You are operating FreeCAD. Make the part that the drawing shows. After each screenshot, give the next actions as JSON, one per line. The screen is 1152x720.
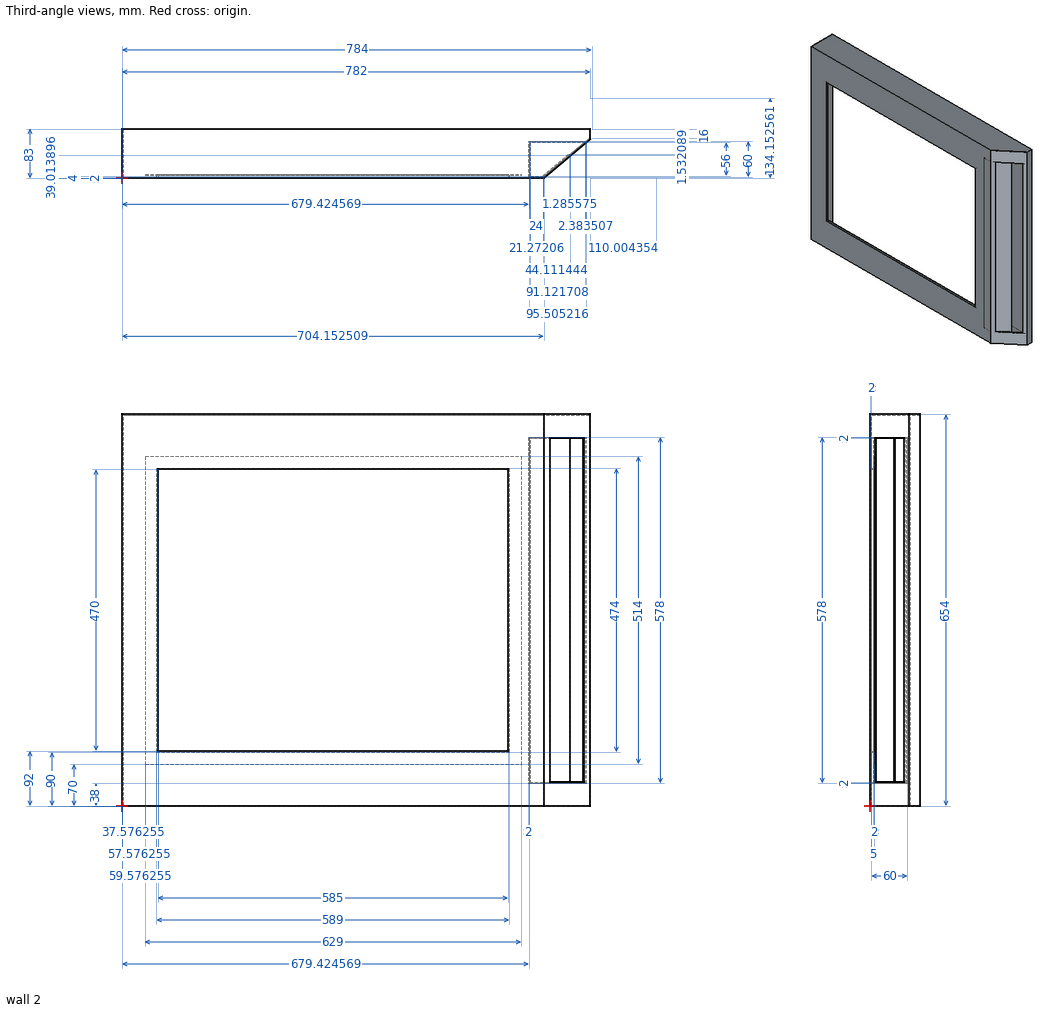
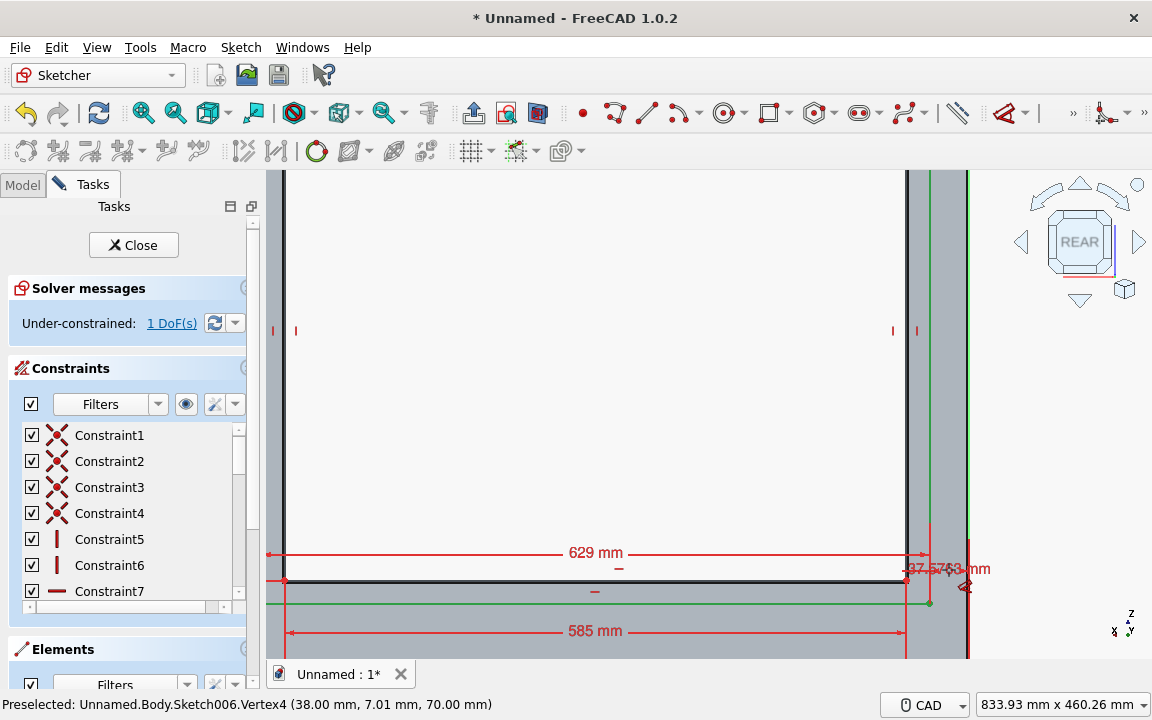
{"action": "left_click", "coordinate": [906, 581]}
{"action": "left_click", "coordinate": [952, 547]}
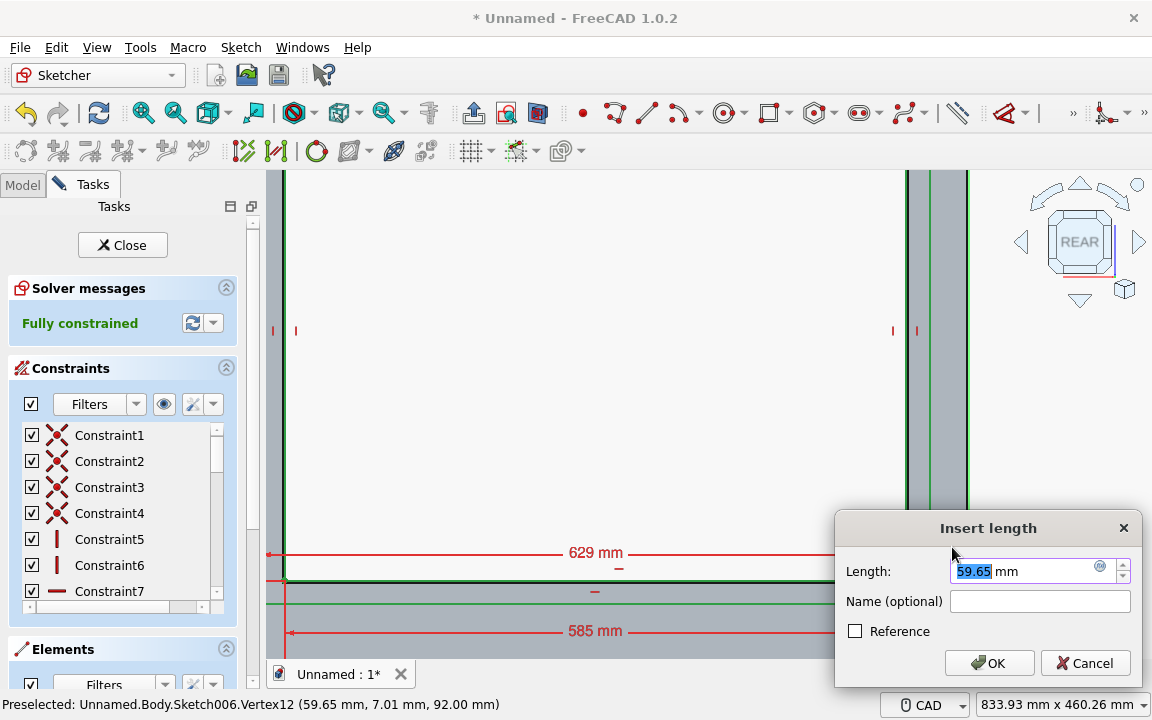
{"action": "type", "text": "59.576255"}
{"action": "key", "text": "Return"}
{"action": "key", "text": "Escape"}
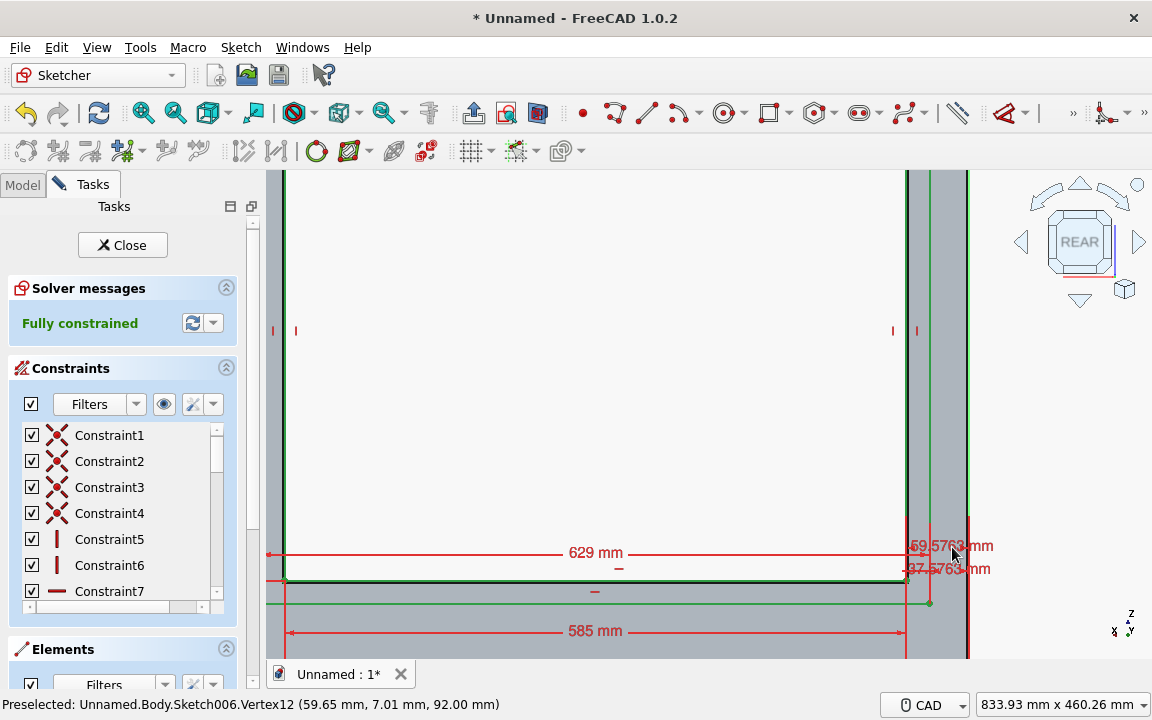
{"action": "left_click", "coordinate": [123, 245]}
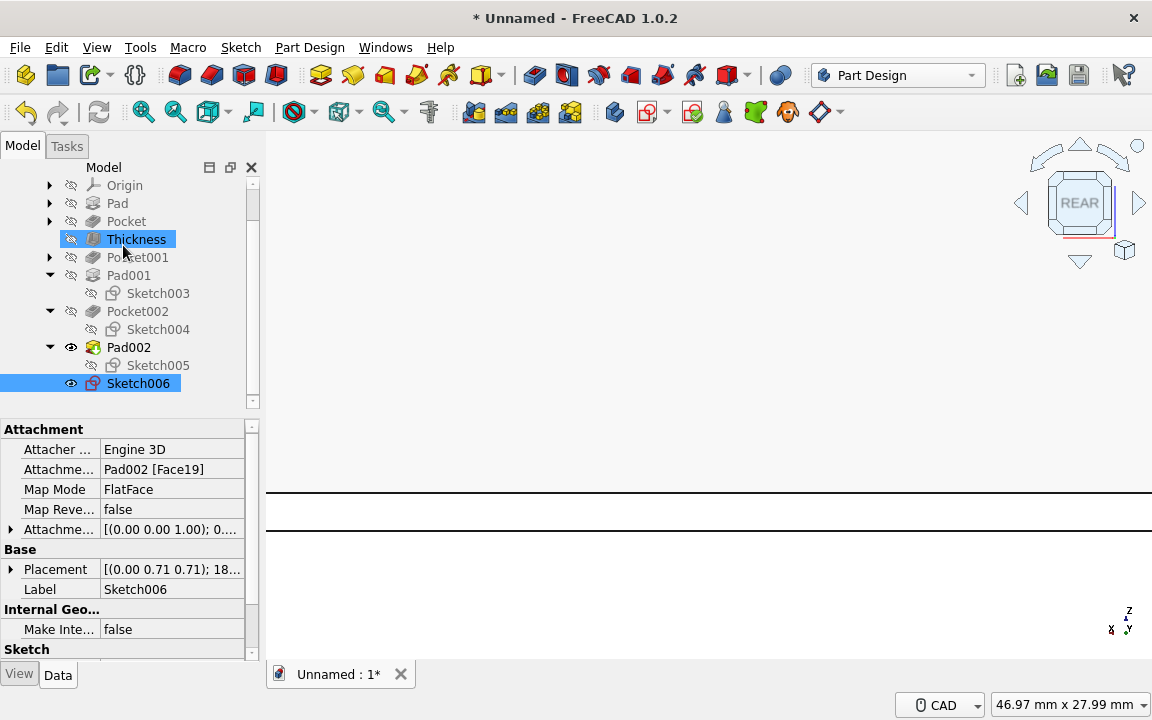
{"action": "left_click", "coordinate": [322, 76]}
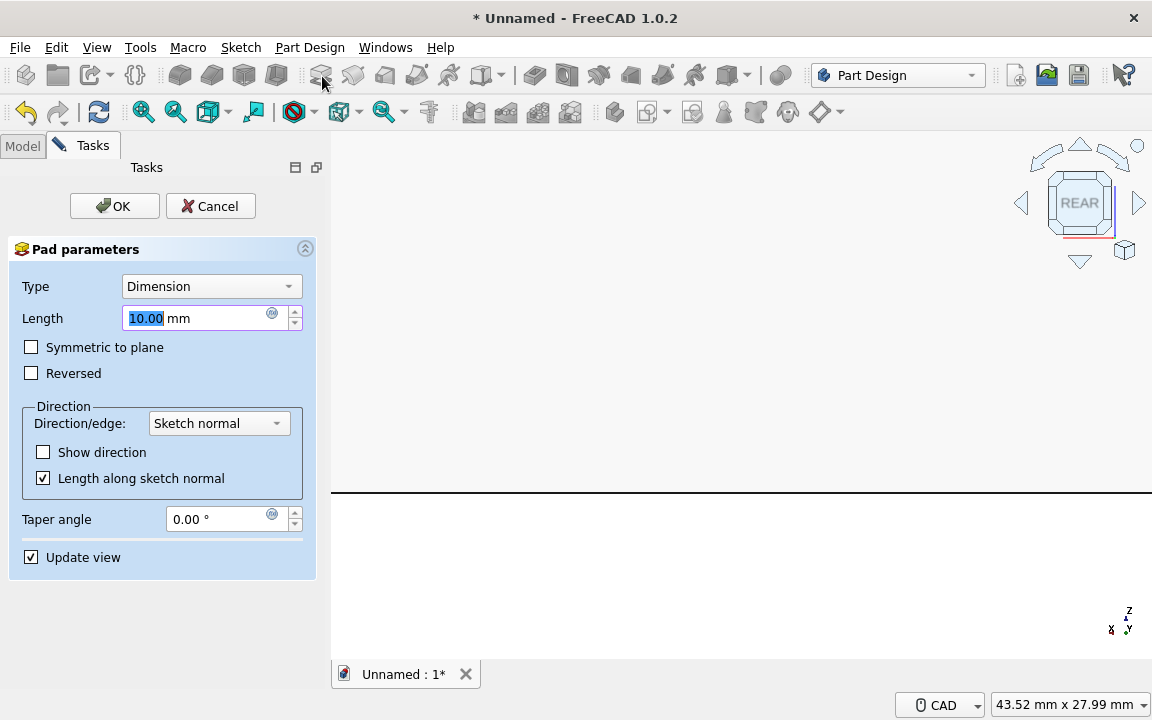
{"action": "type", "text": "2"}
{"action": "key", "text": "Tab"}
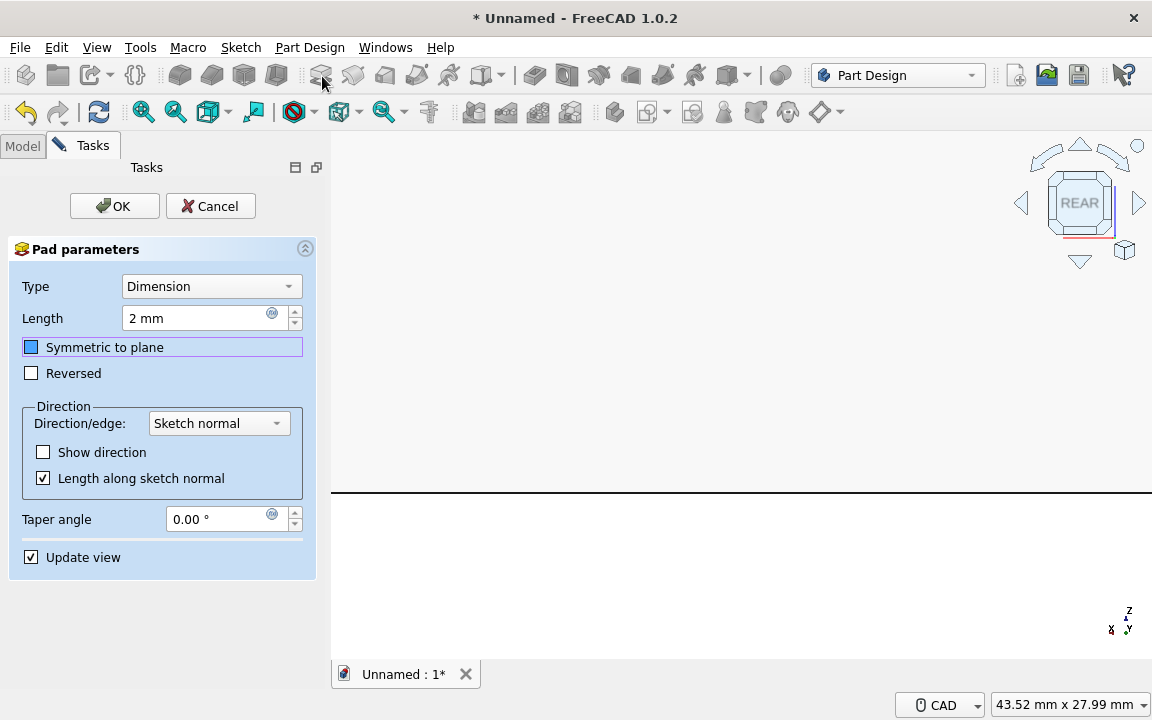
{"action": "left_click", "coordinate": [30, 373]}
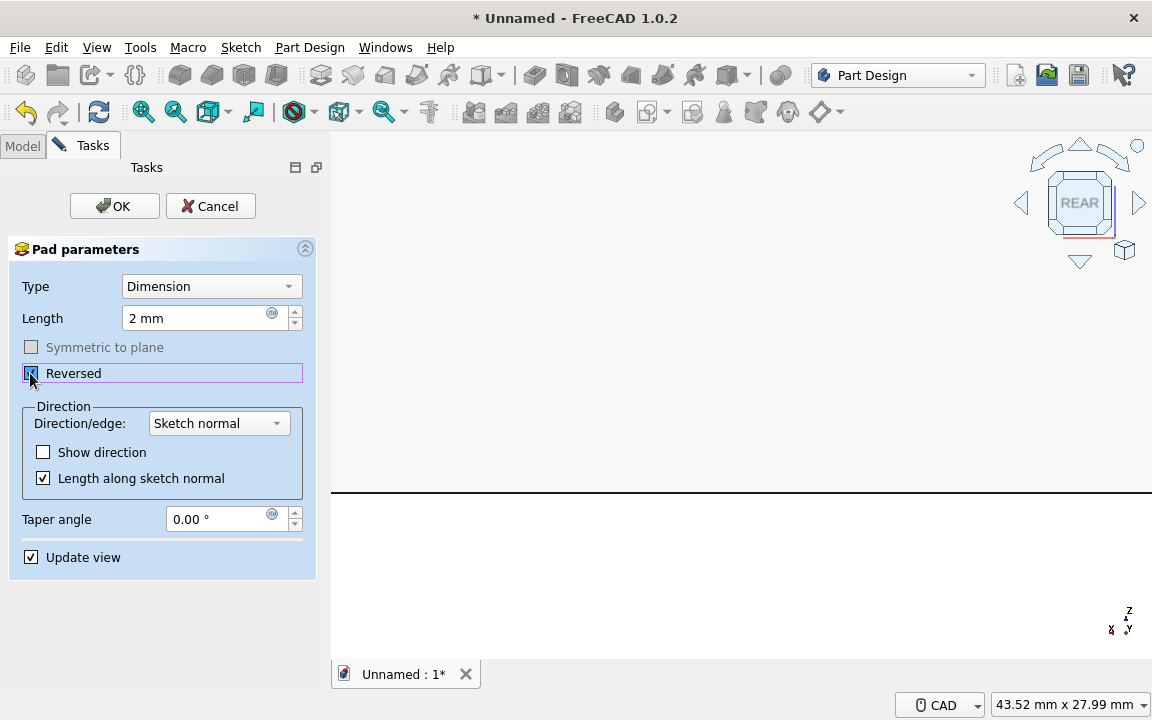
{"action": "left_click", "coordinate": [115, 206]}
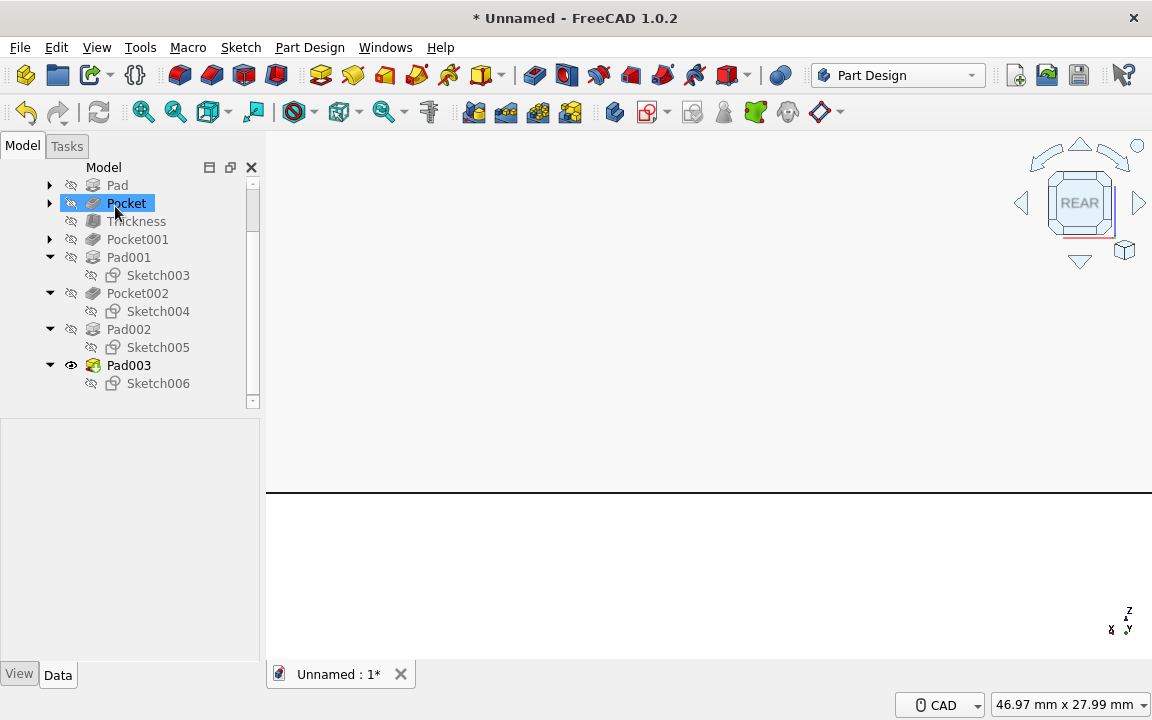
{"action": "left_click", "coordinate": [144, 112]}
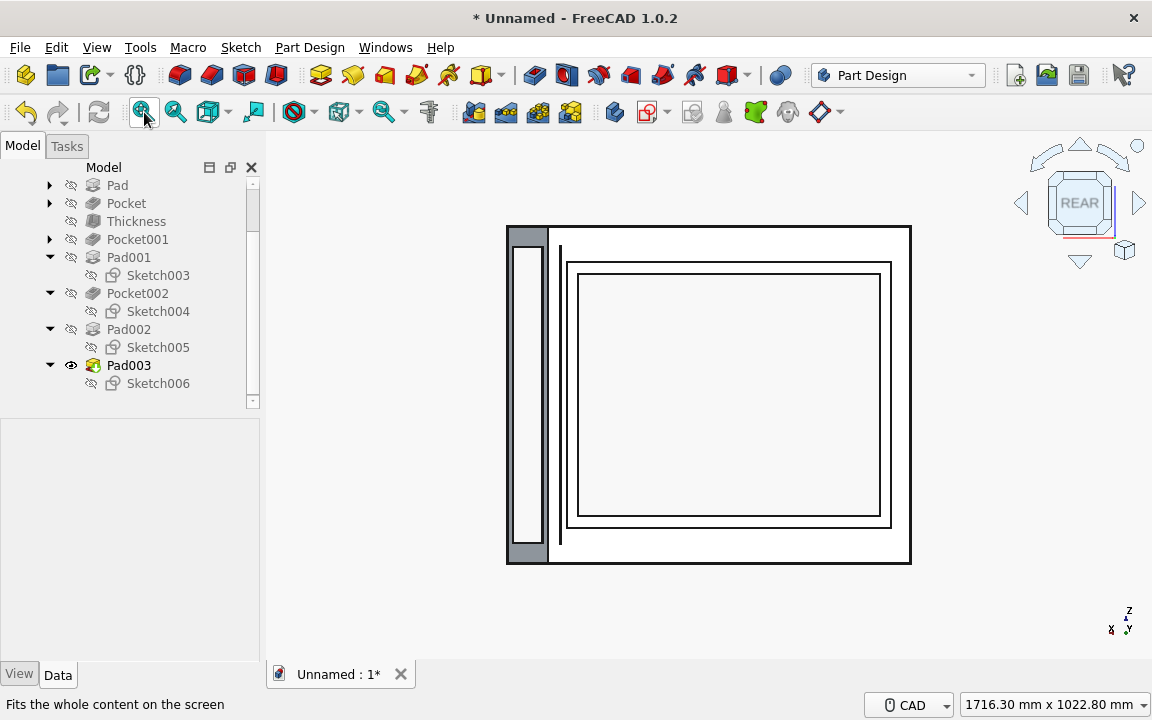
{"action": "left_click", "coordinate": [616, 112]}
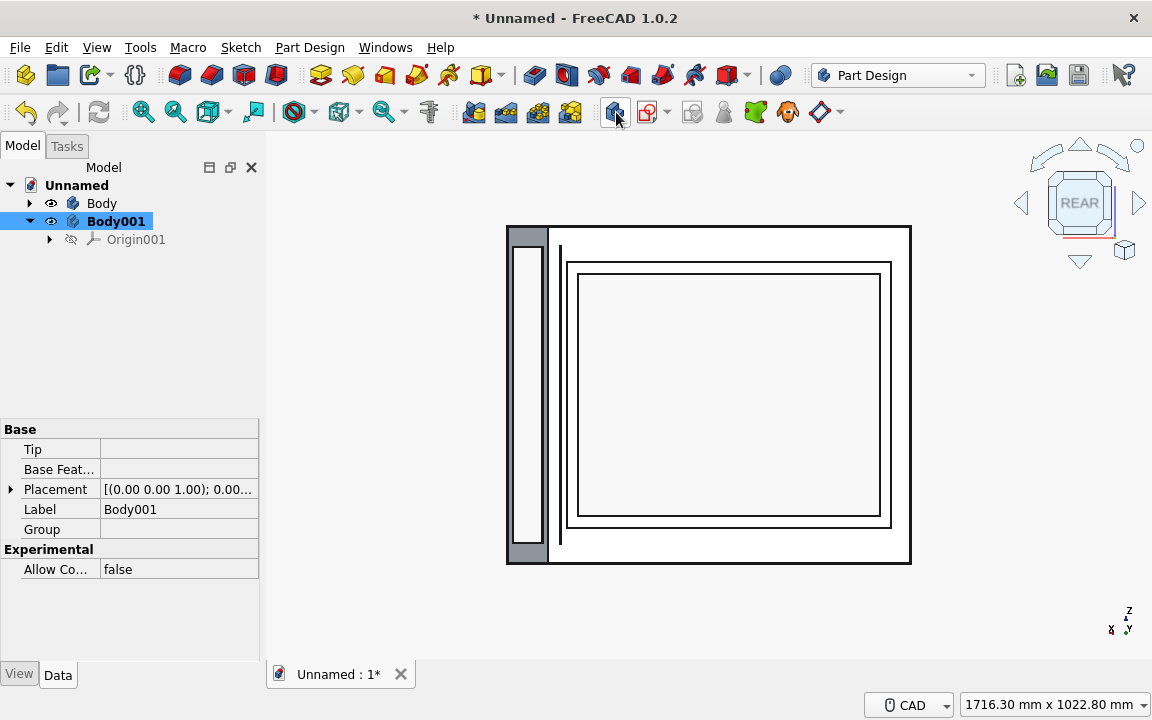
{"action": "left_click", "coordinate": [50, 239]}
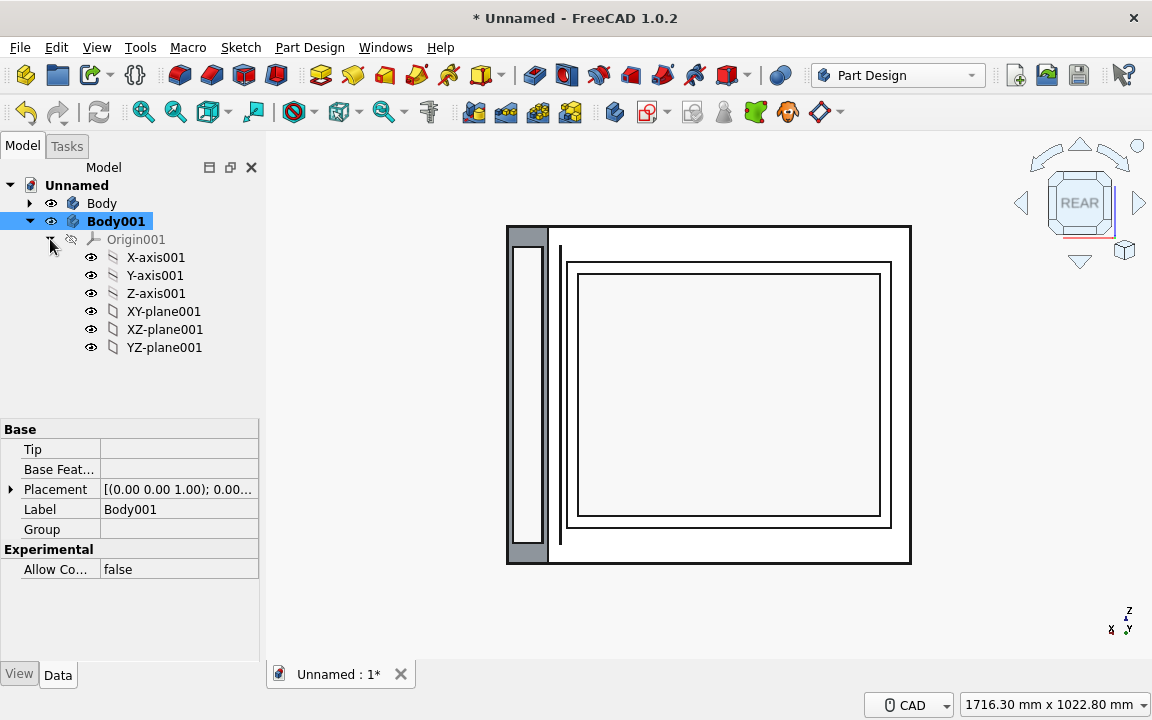
{"action": "left_click", "coordinate": [136, 311]}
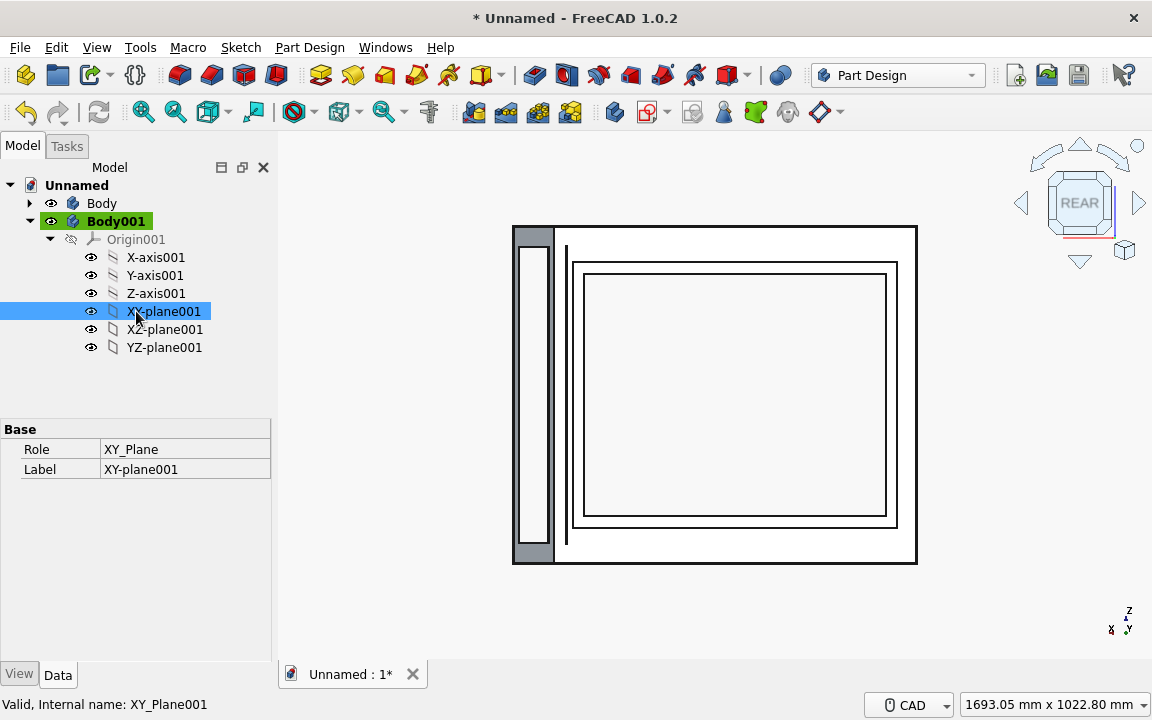
{"action": "left_click", "coordinate": [820, 112]}